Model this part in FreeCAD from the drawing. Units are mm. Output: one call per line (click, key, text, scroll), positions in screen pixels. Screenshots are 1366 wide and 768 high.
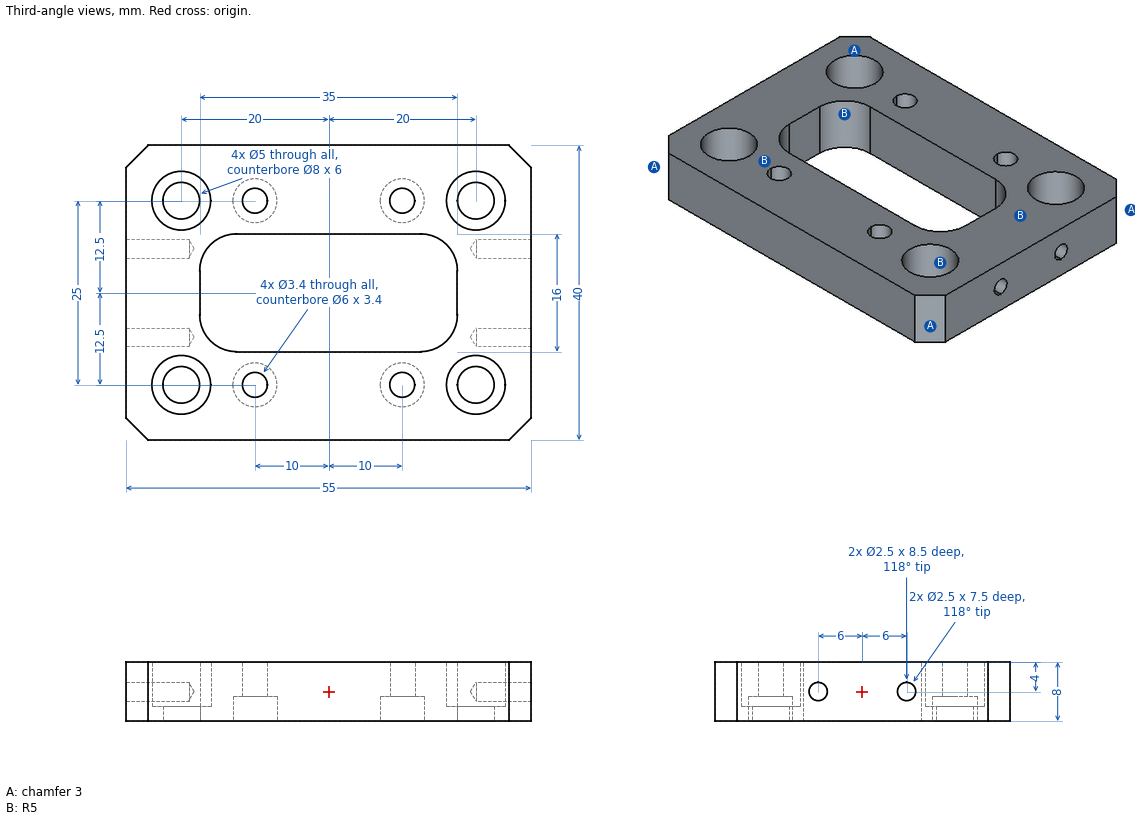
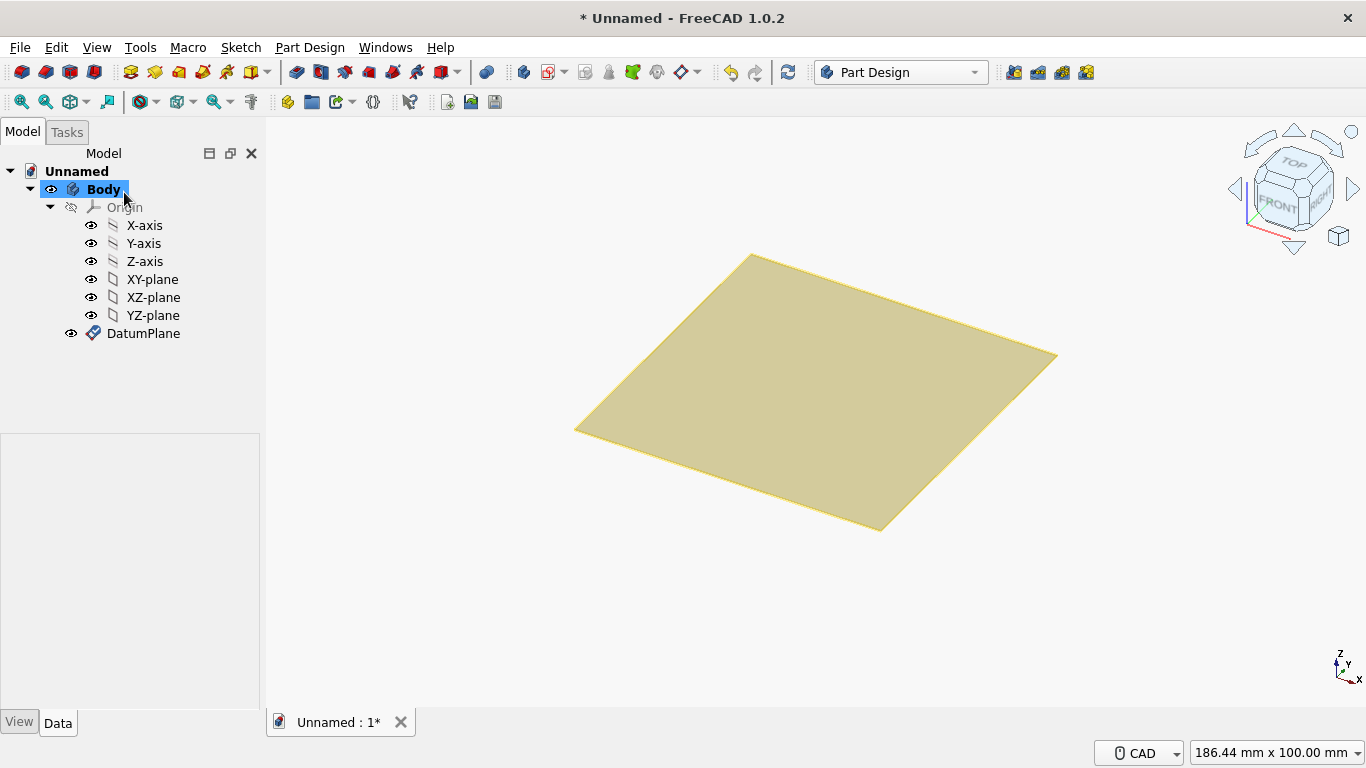
click(116, 333)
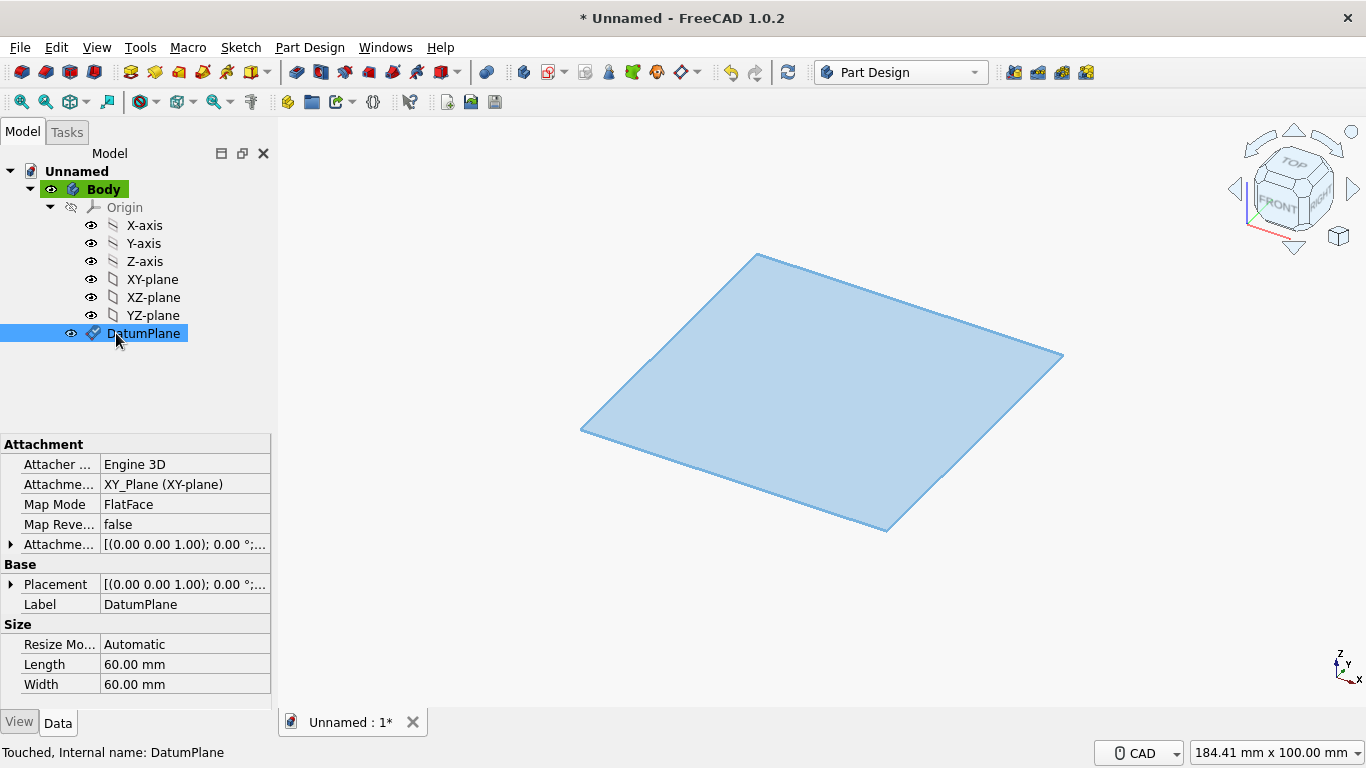
click(548, 72)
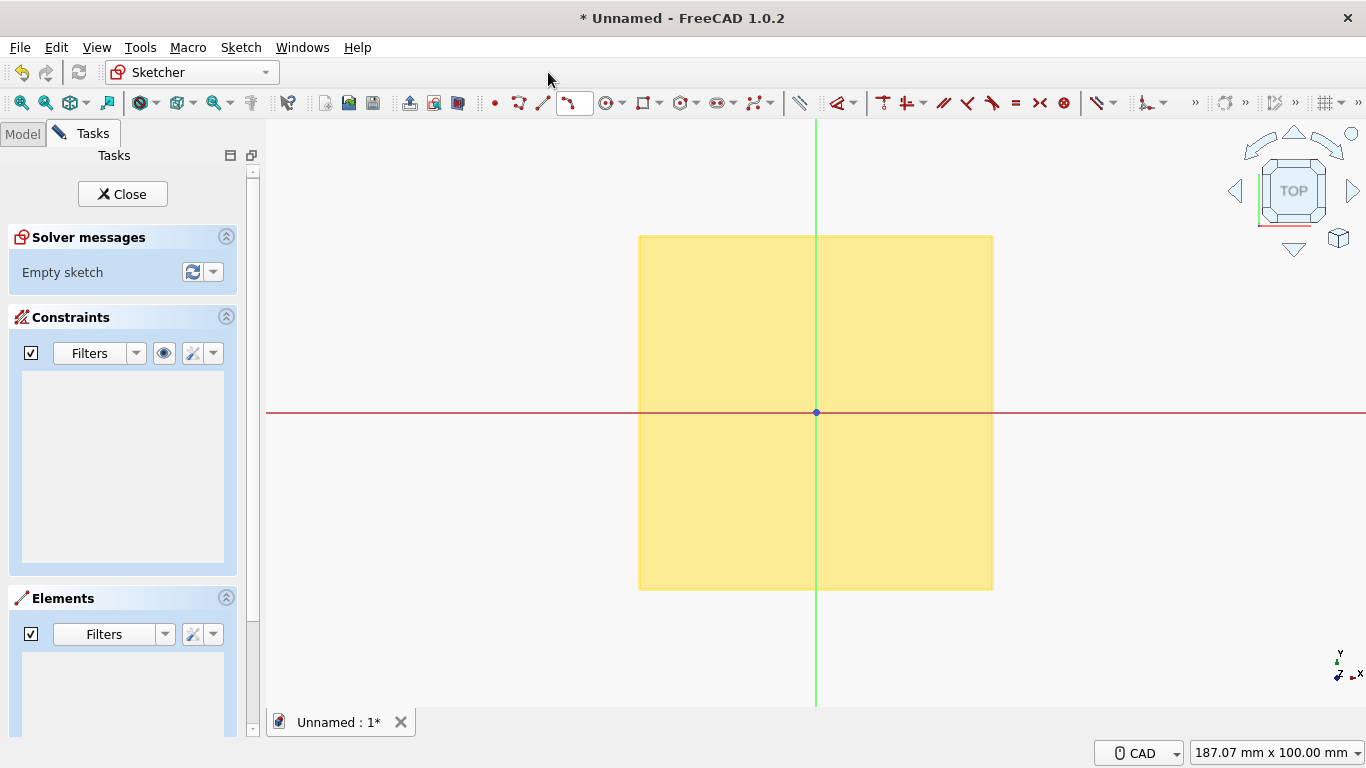
scroll(955, 413, up, 2)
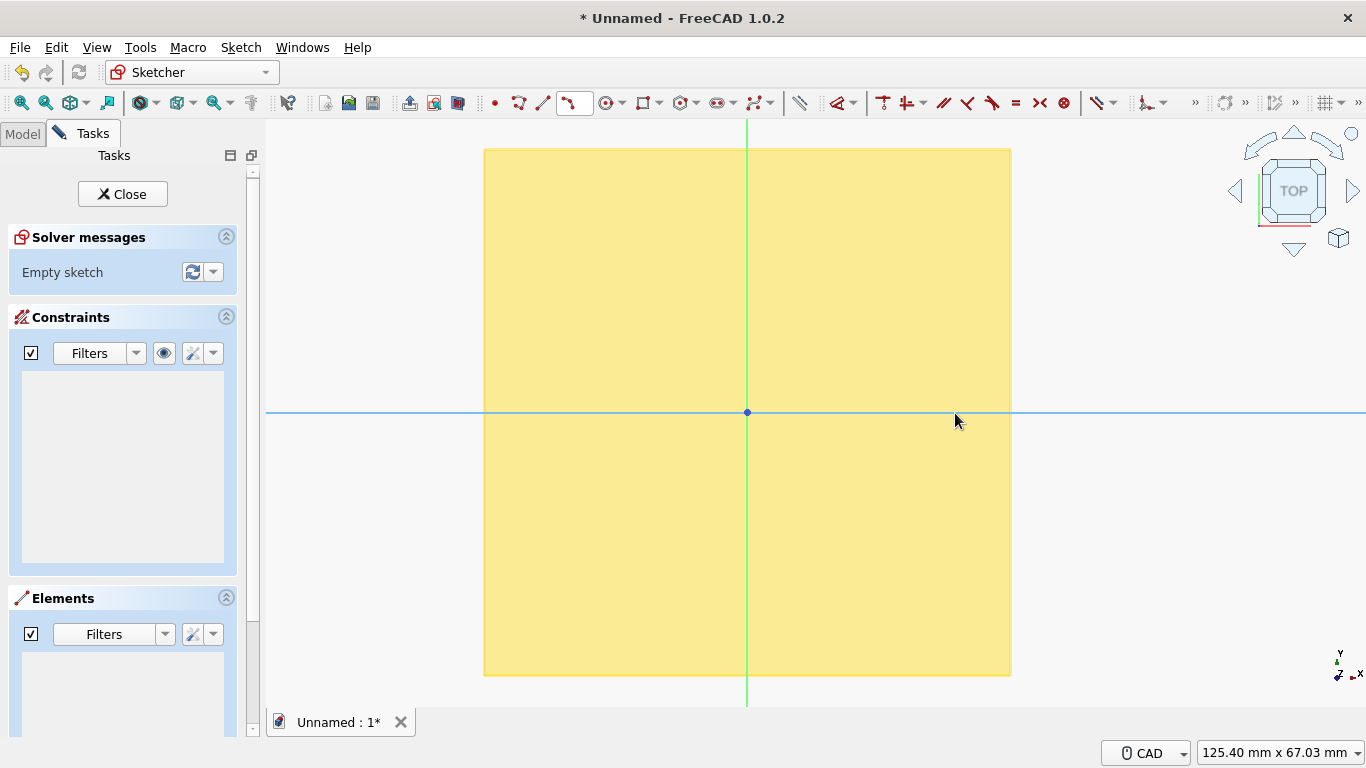
key(g)
key(v)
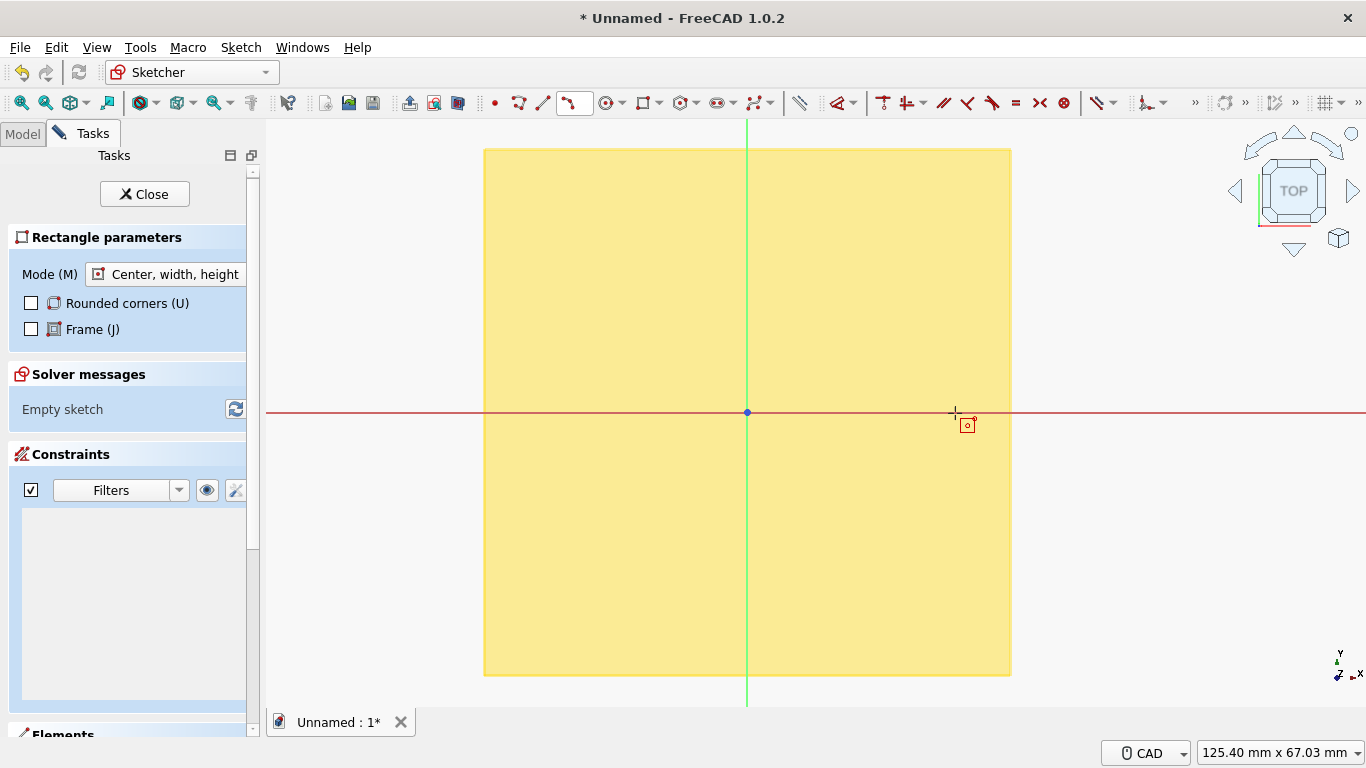
click(747, 413)
move(989, 237)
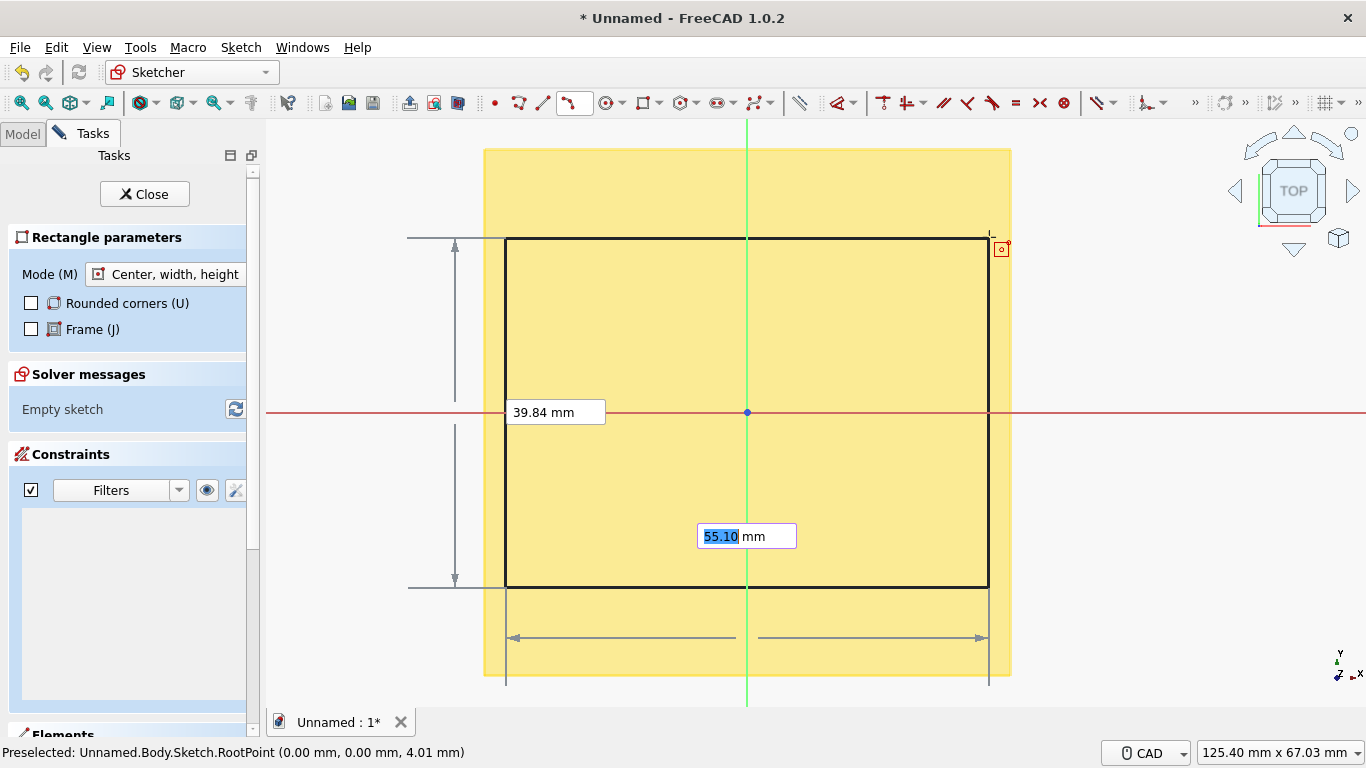
text(55)
key(Tab)
text(40)
key(Return)
key(Escape)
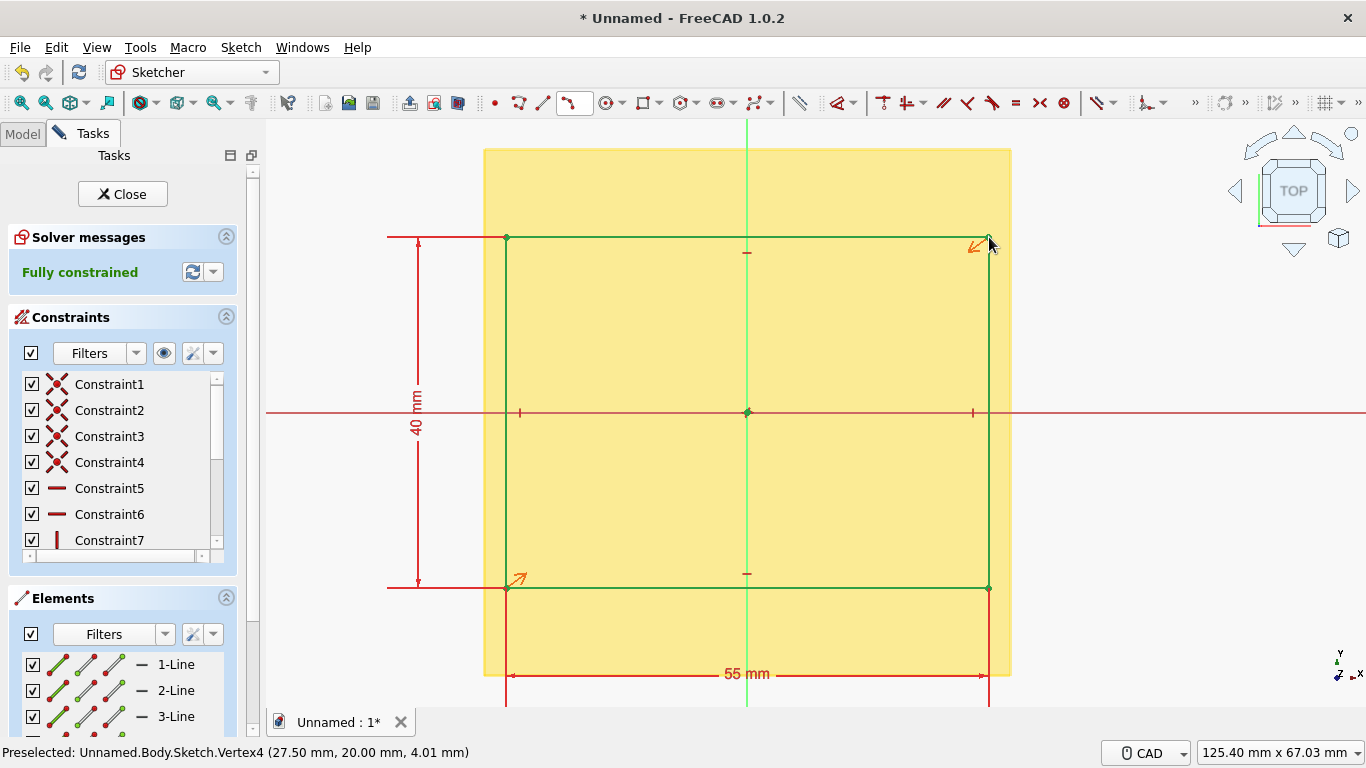
click(123, 194)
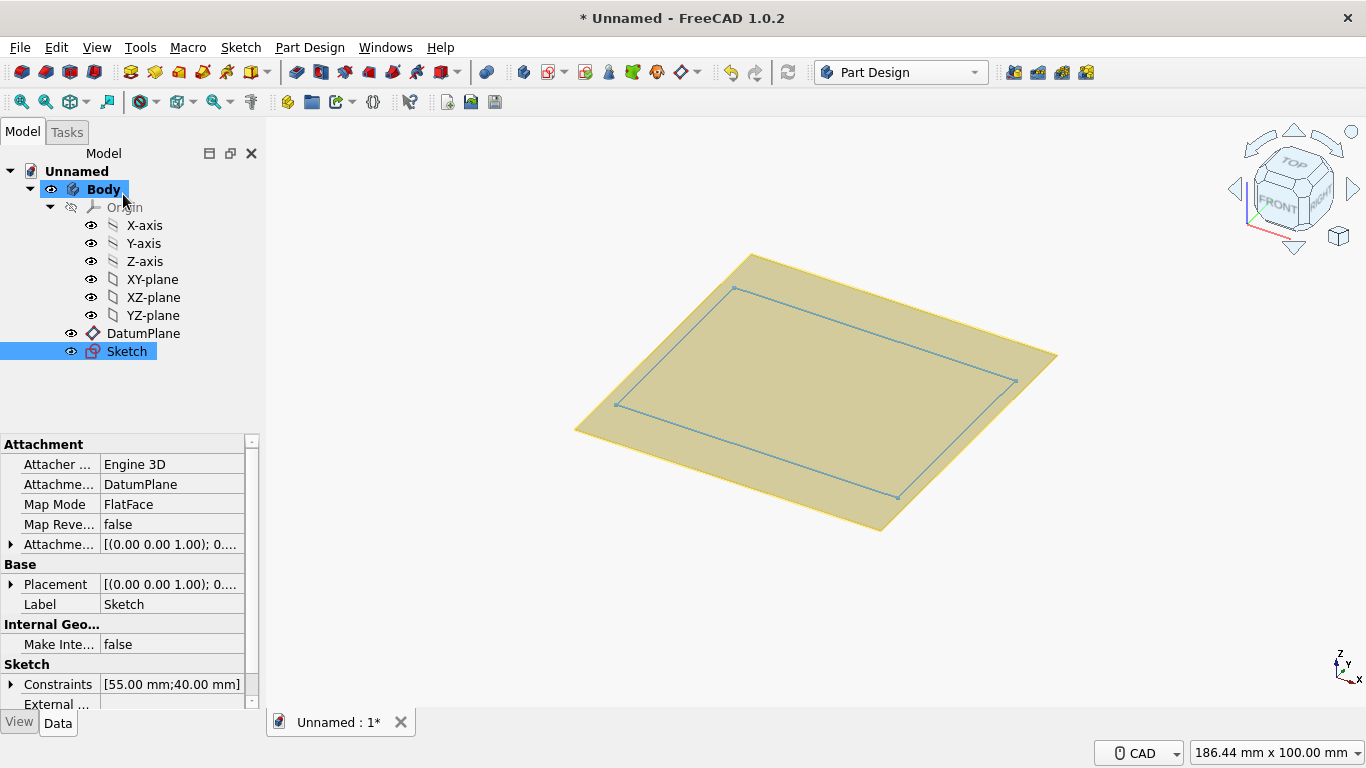
click(132, 72)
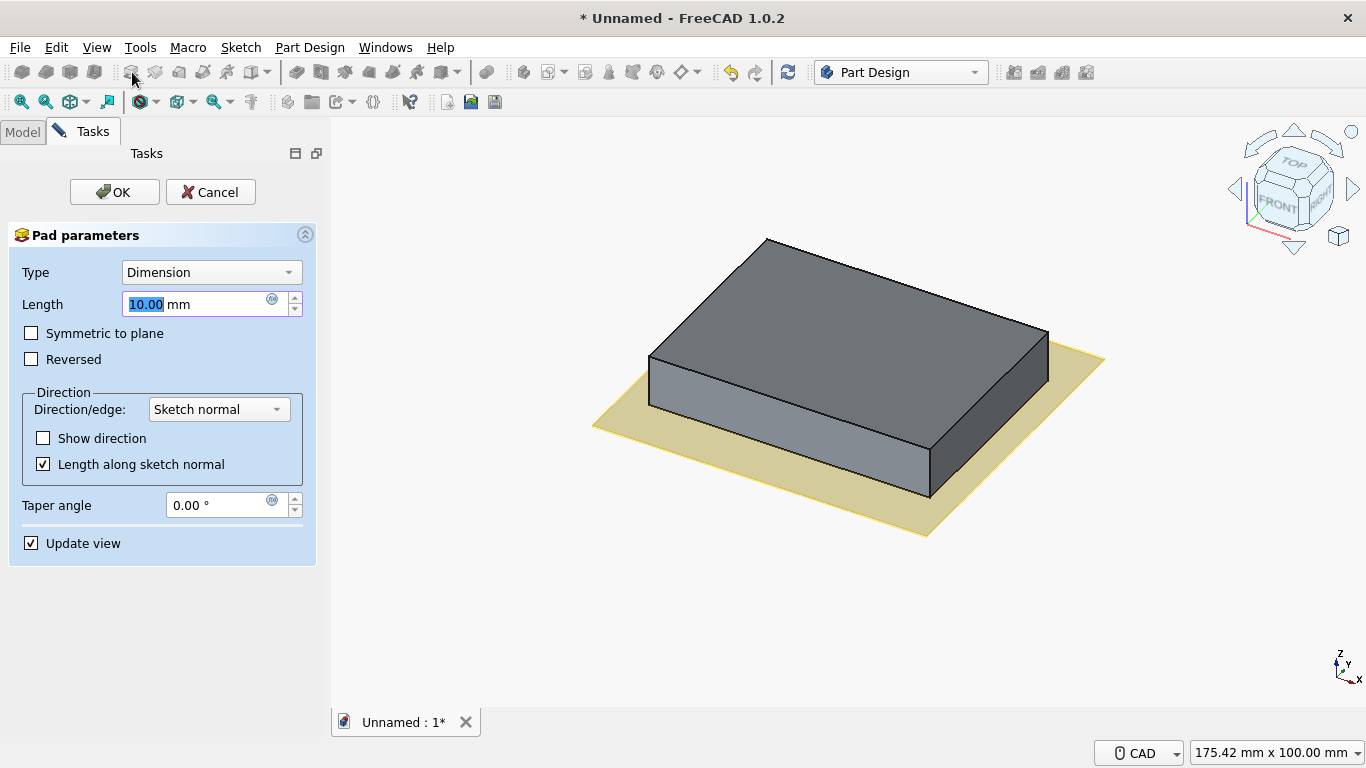
text(8)
key(Tab)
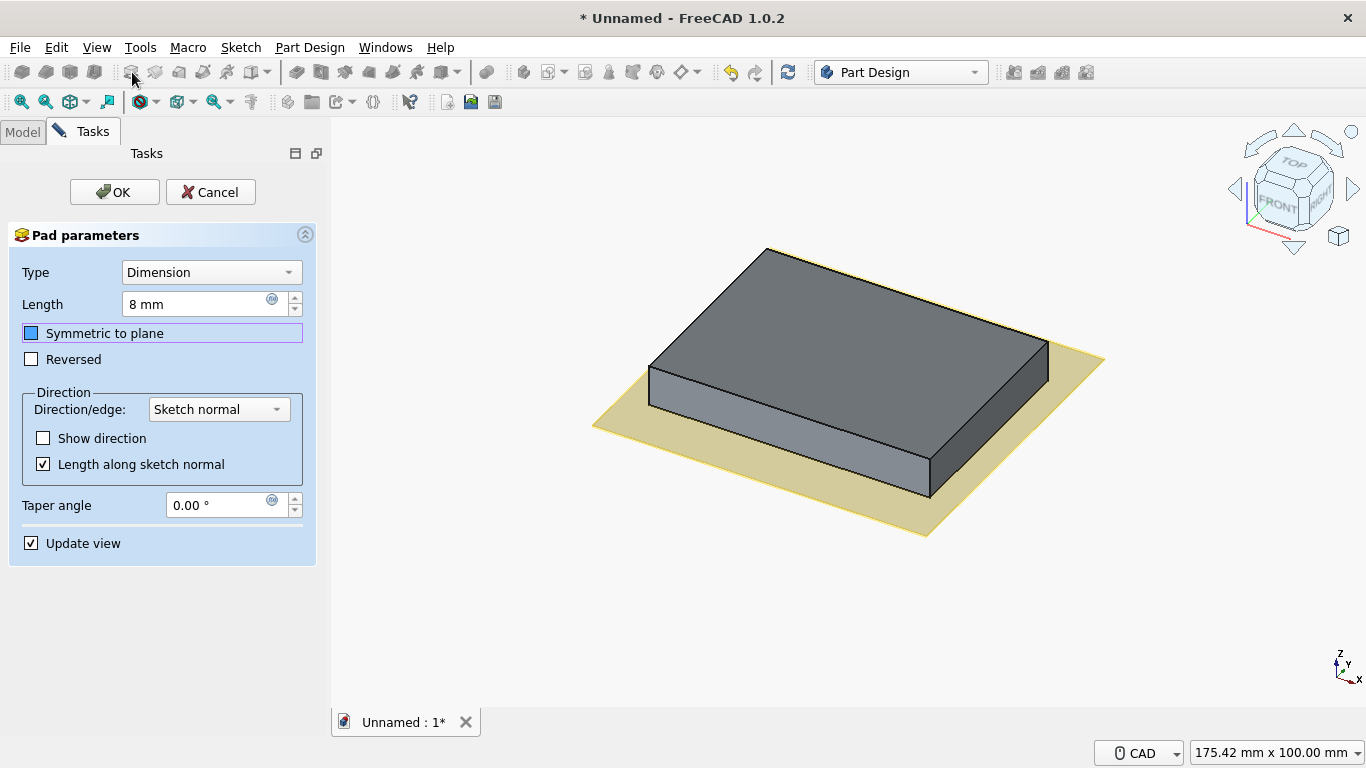
click(30, 359)